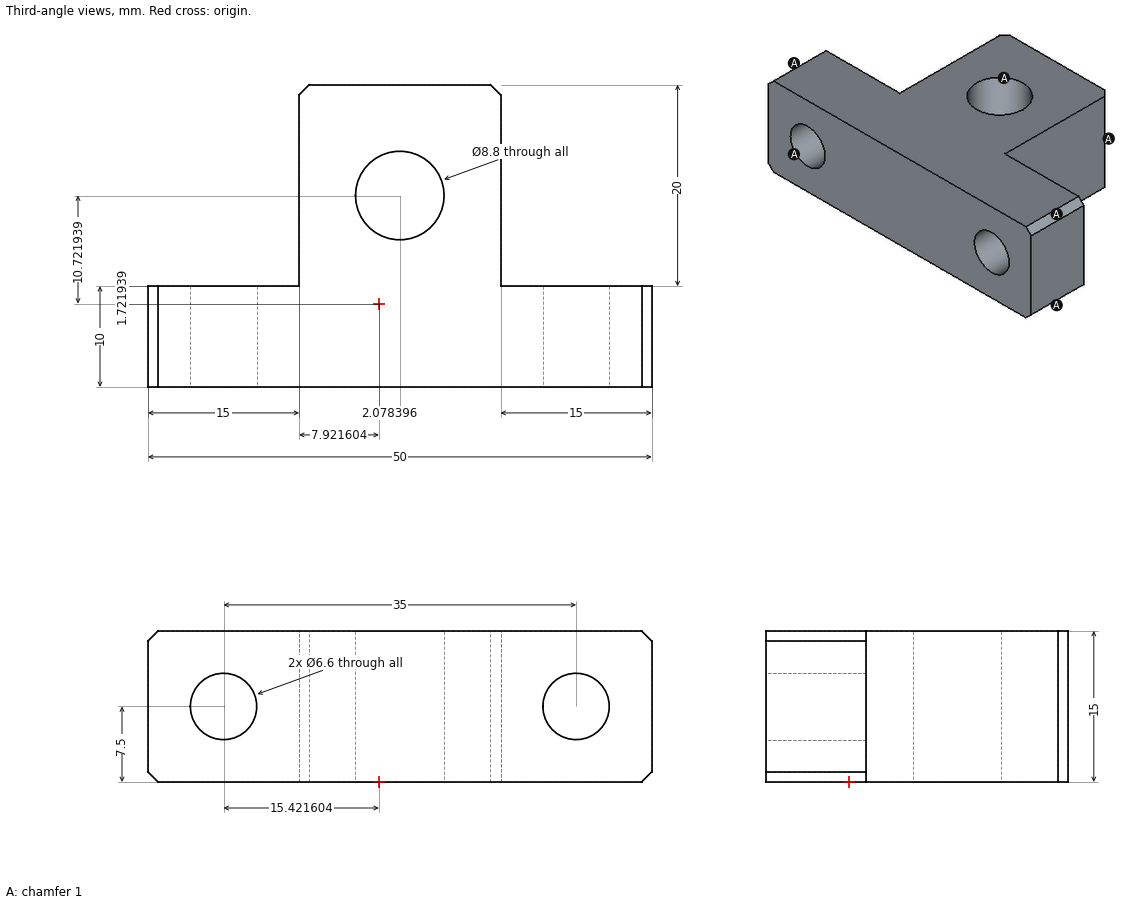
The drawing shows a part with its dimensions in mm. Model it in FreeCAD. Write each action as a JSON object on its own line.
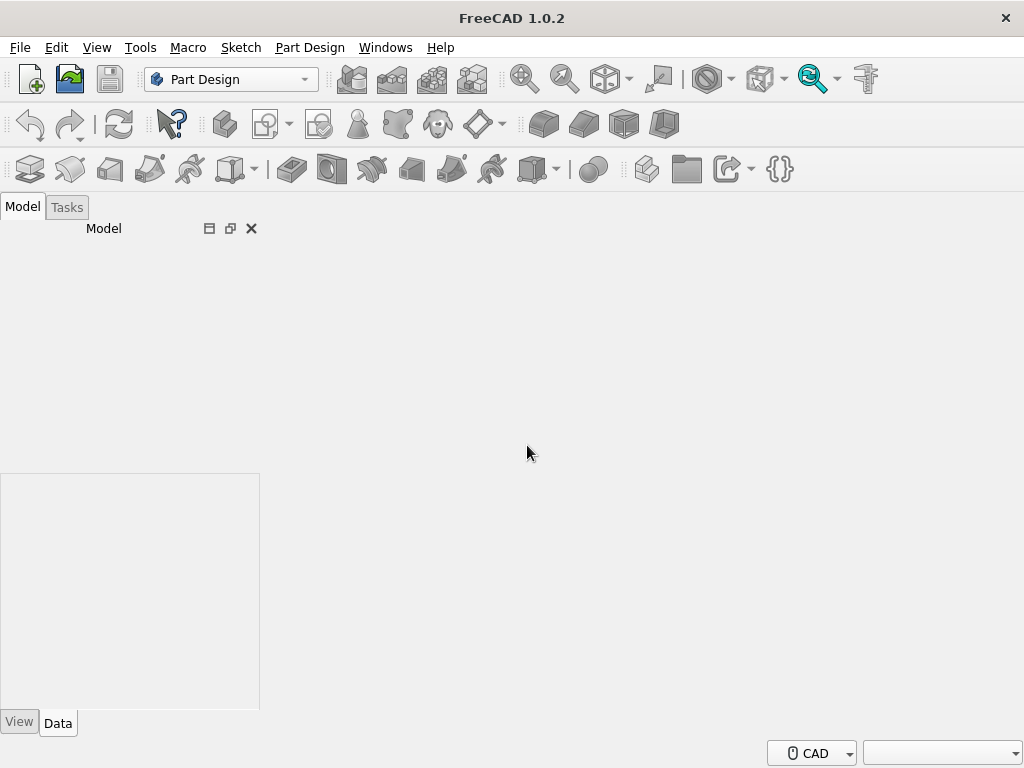
{"action": "left_click", "coordinate": [30, 80]}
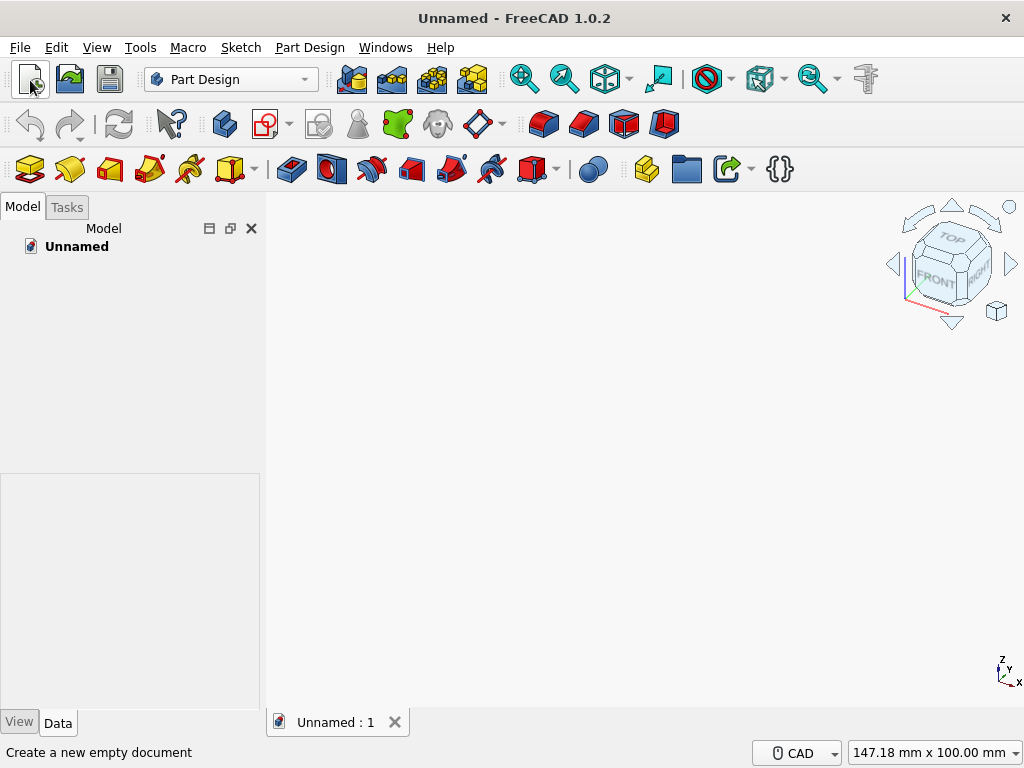
{"action": "left_click", "coordinate": [266, 124]}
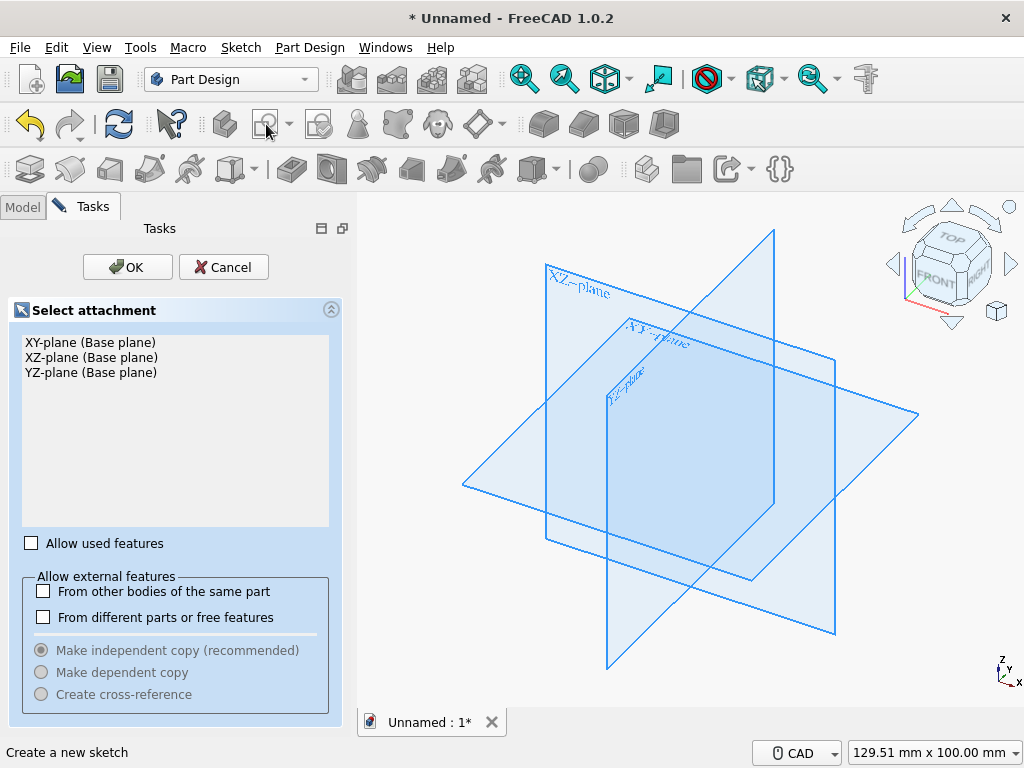
{"action": "left_click", "coordinate": [82, 342]}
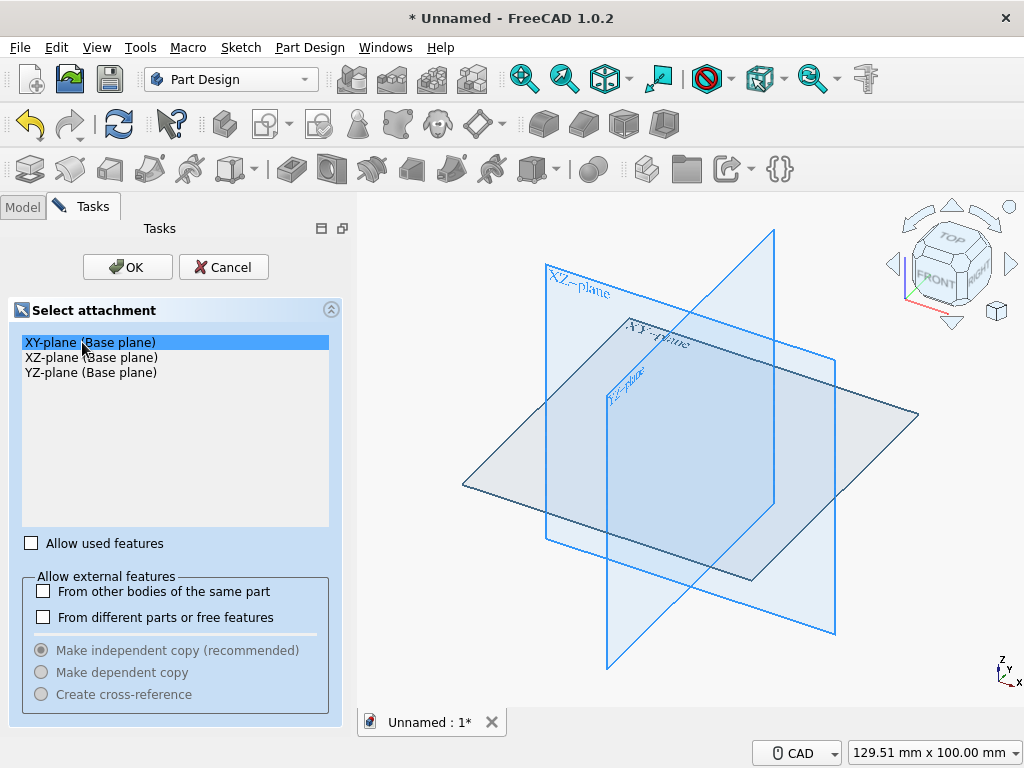
{"action": "left_click", "coordinate": [128, 267]}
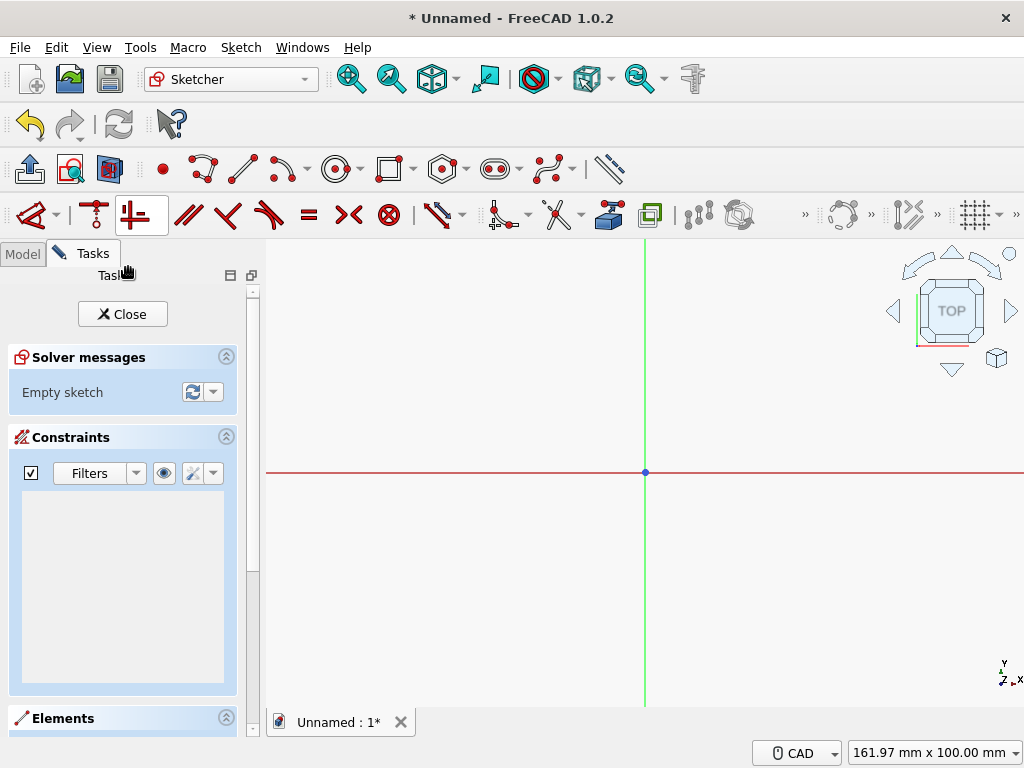
{"action": "scroll", "coordinate": [750, 403], "scroll_direction": "up", "scroll_amount": 3}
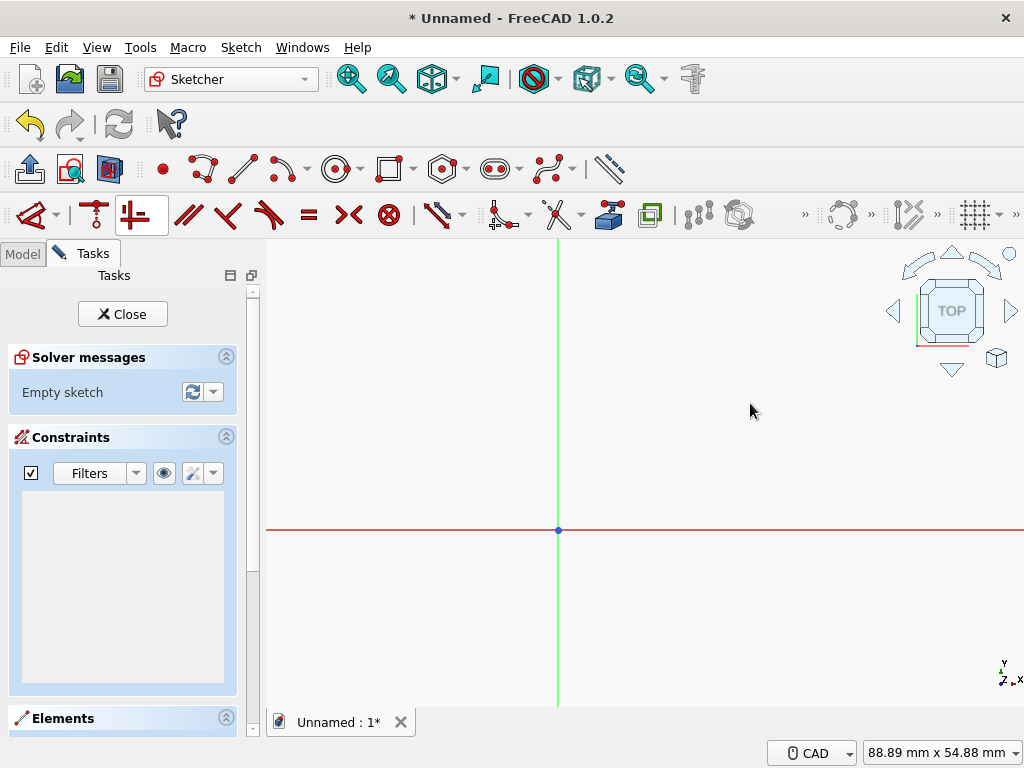
{"action": "left_click", "coordinate": [204, 170]}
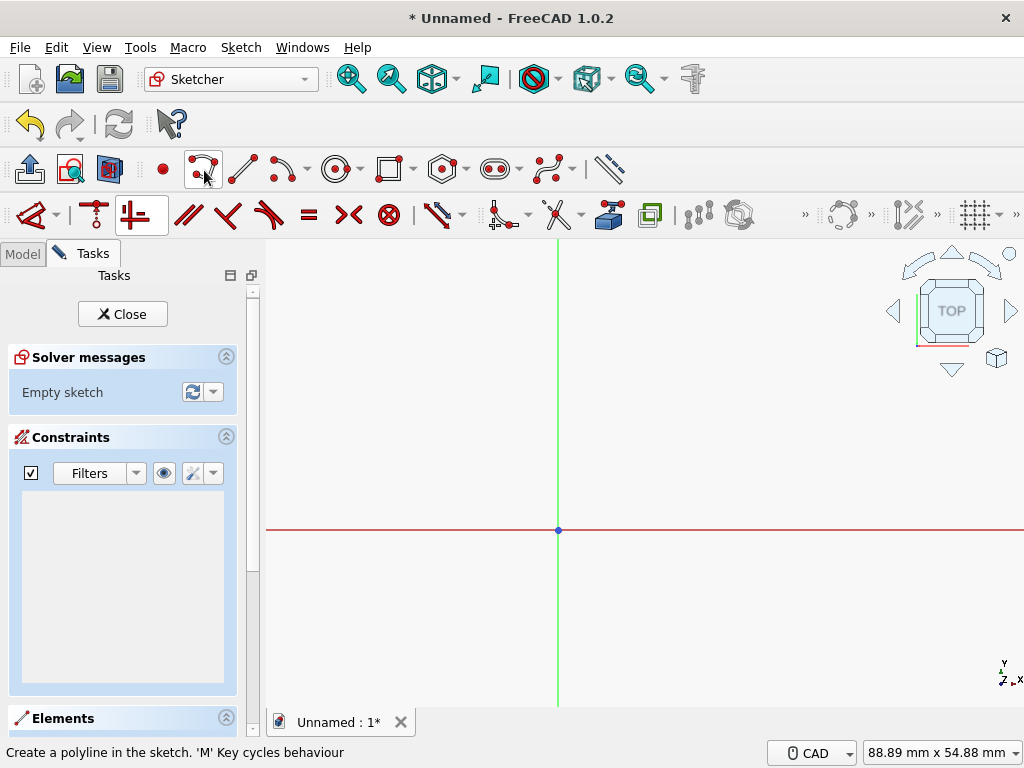
{"action": "left_click", "coordinate": [491, 516]}
{"action": "left_click", "coordinate": [363, 516]}
{"action": "left_click", "coordinate": [363, 601]}
{"action": "left_click", "coordinate": [789, 601]}
{"action": "left_click", "coordinate": [789, 516]}
{"action": "left_click", "coordinate": [661, 516]}
{"action": "left_click", "coordinate": [661, 345]}
{"action": "left_click", "coordinate": [491, 345]}
{"action": "left_click", "coordinate": [491, 517]}
{"action": "key", "text": "Escape"}
{"action": "key", "text": "Escape"}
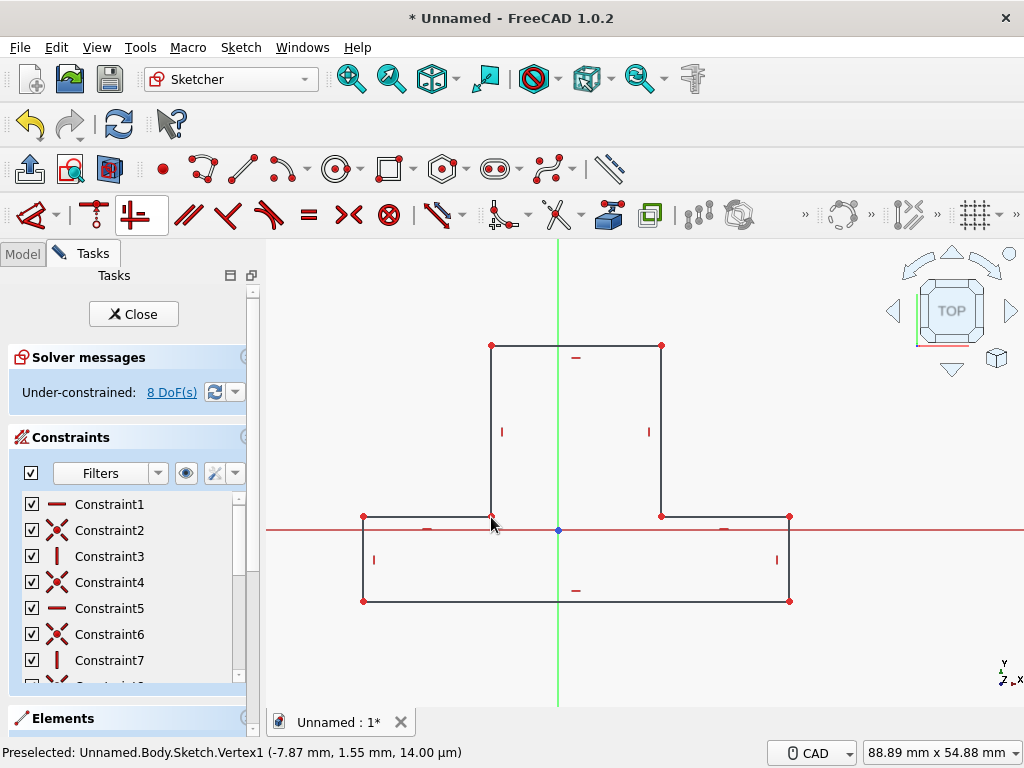
{"action": "left_click", "coordinate": [453, 517]}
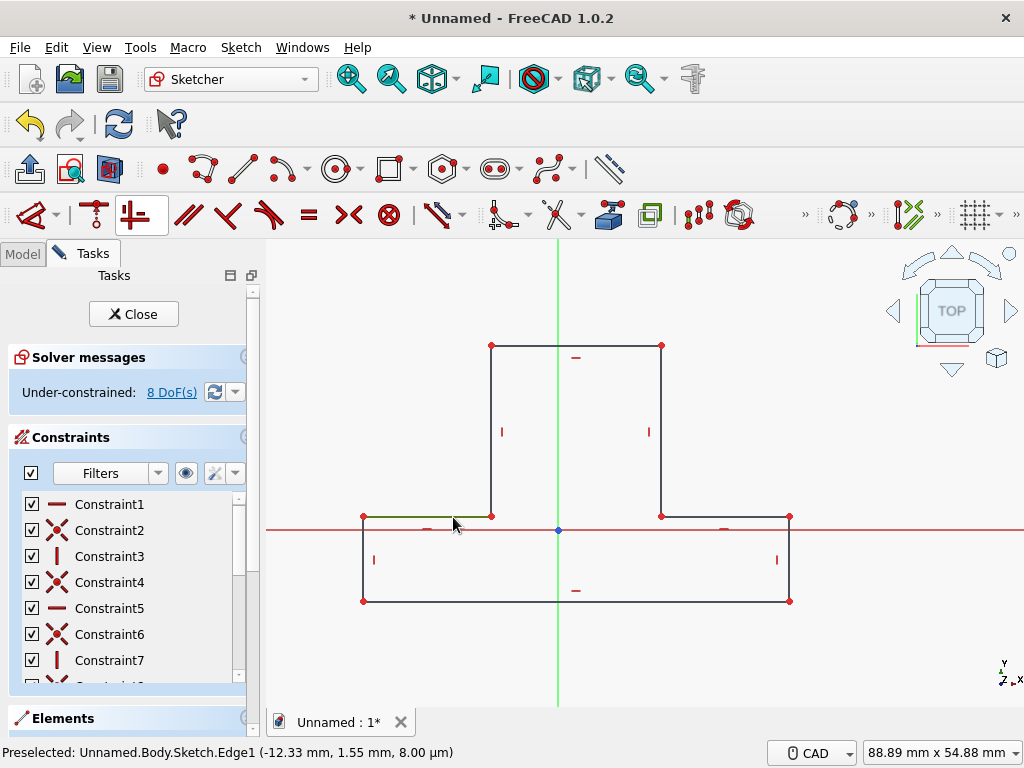
{"action": "key", "text": "l"}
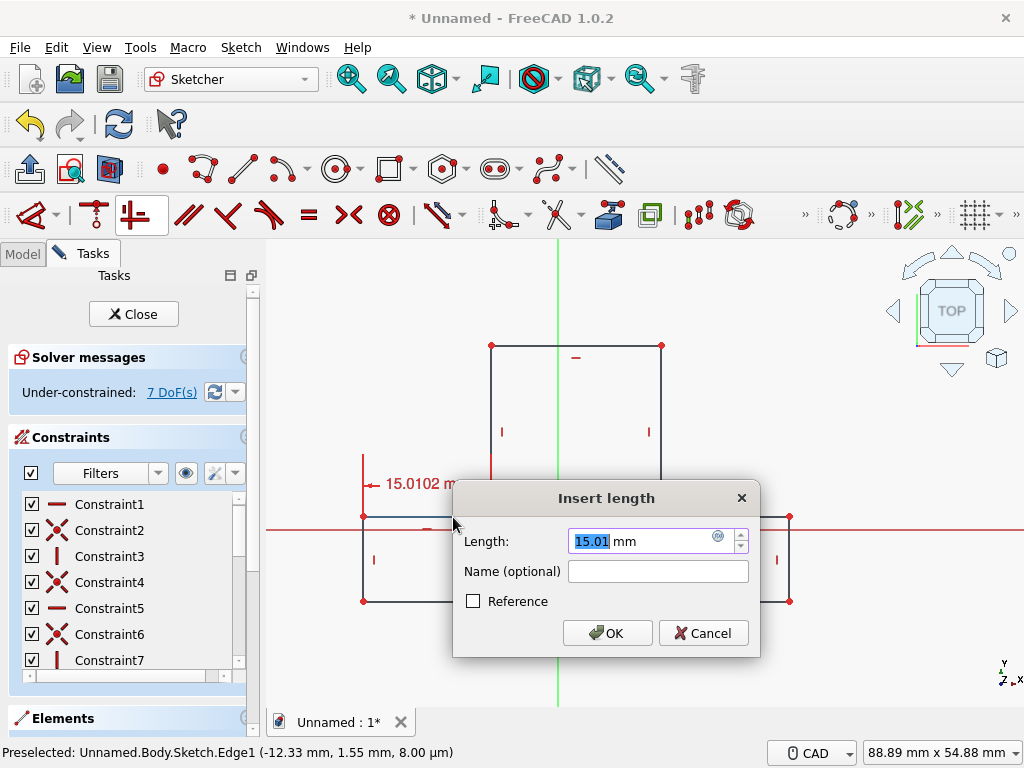
{"action": "type", "text": "15"}
{"action": "key", "text": "Return"}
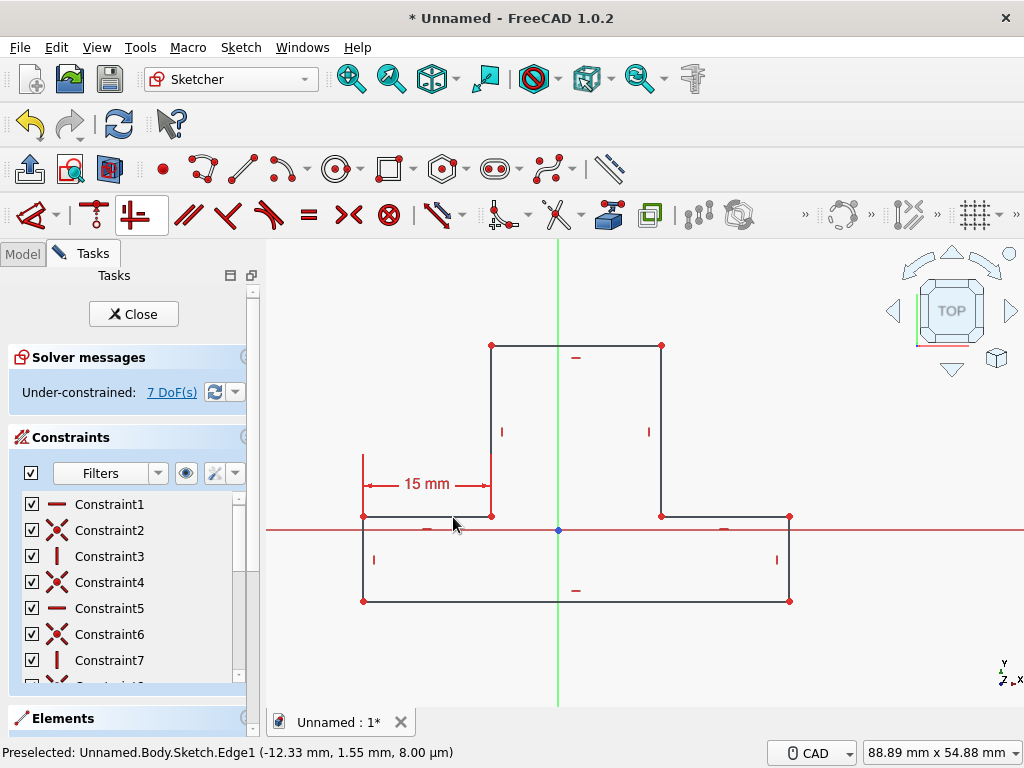
{"action": "left_click", "coordinate": [363, 542]}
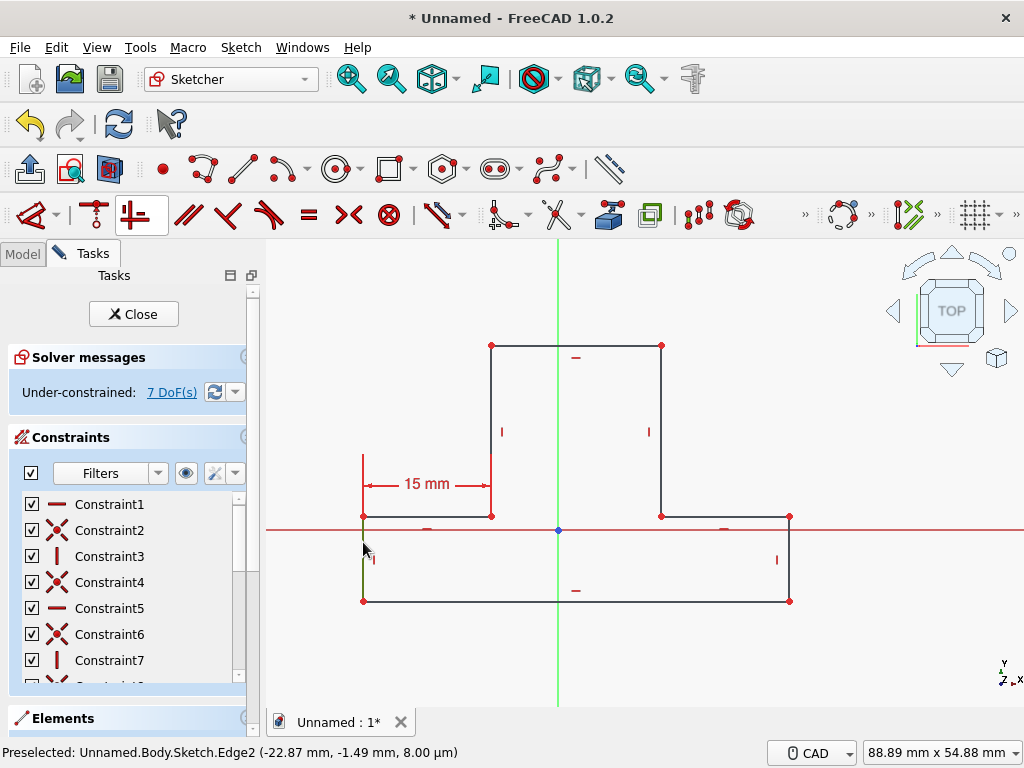
{"action": "left_click", "coordinate": [58, 216]}